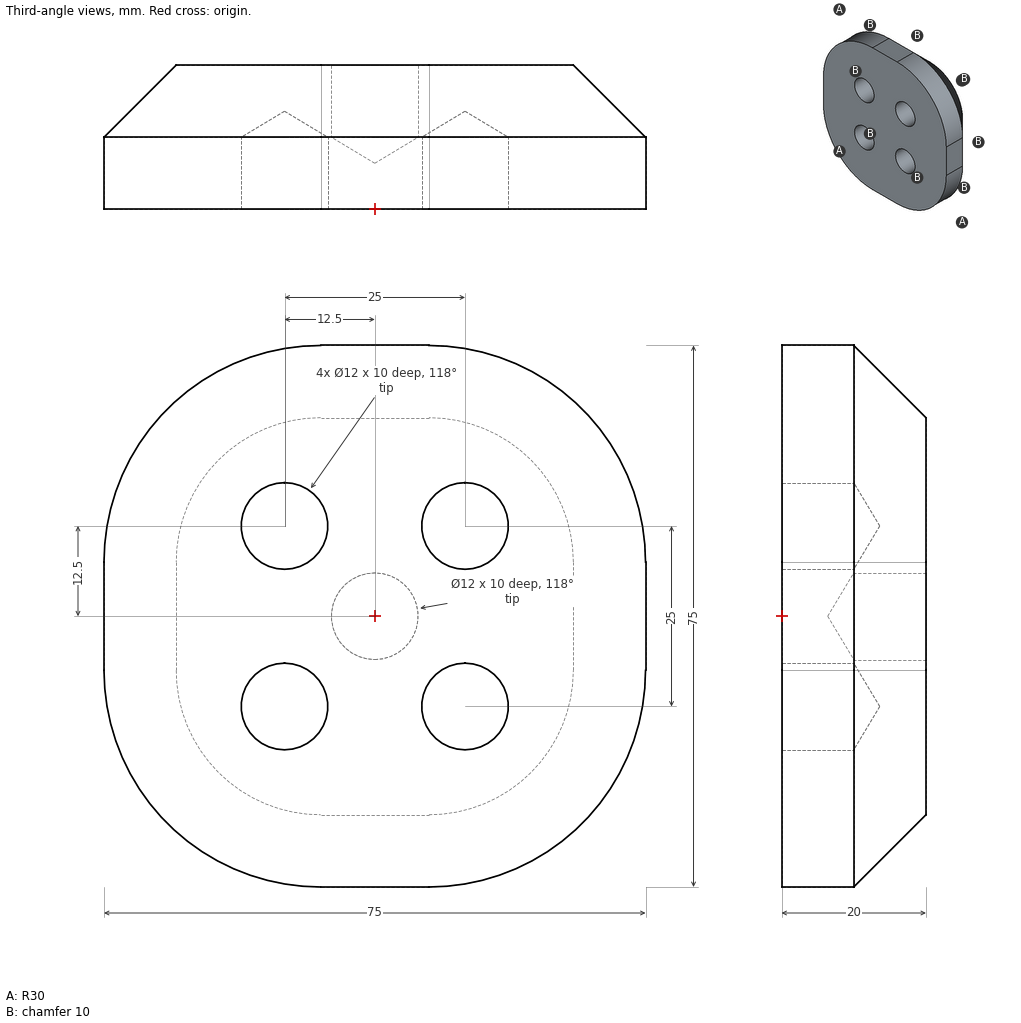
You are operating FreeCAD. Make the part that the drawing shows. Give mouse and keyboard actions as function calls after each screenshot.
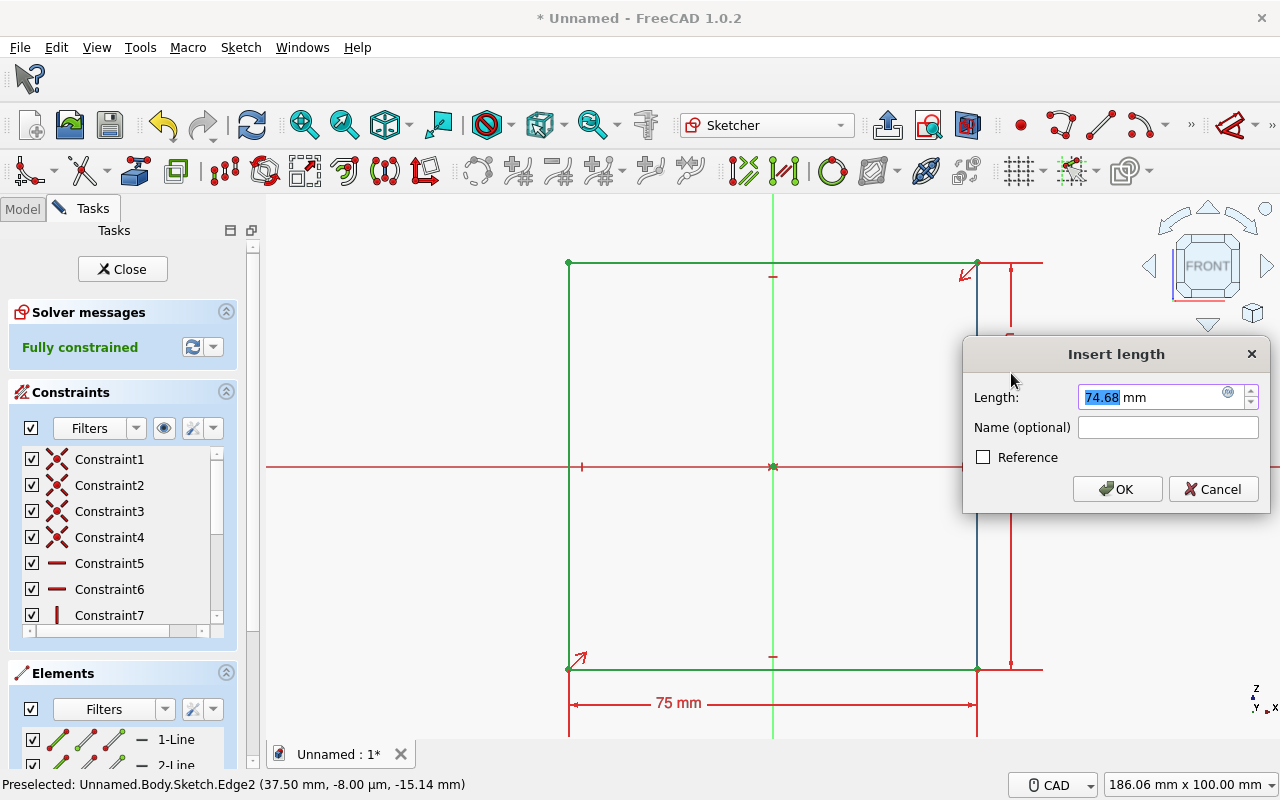
text(75)
key(Return)
key(Escape)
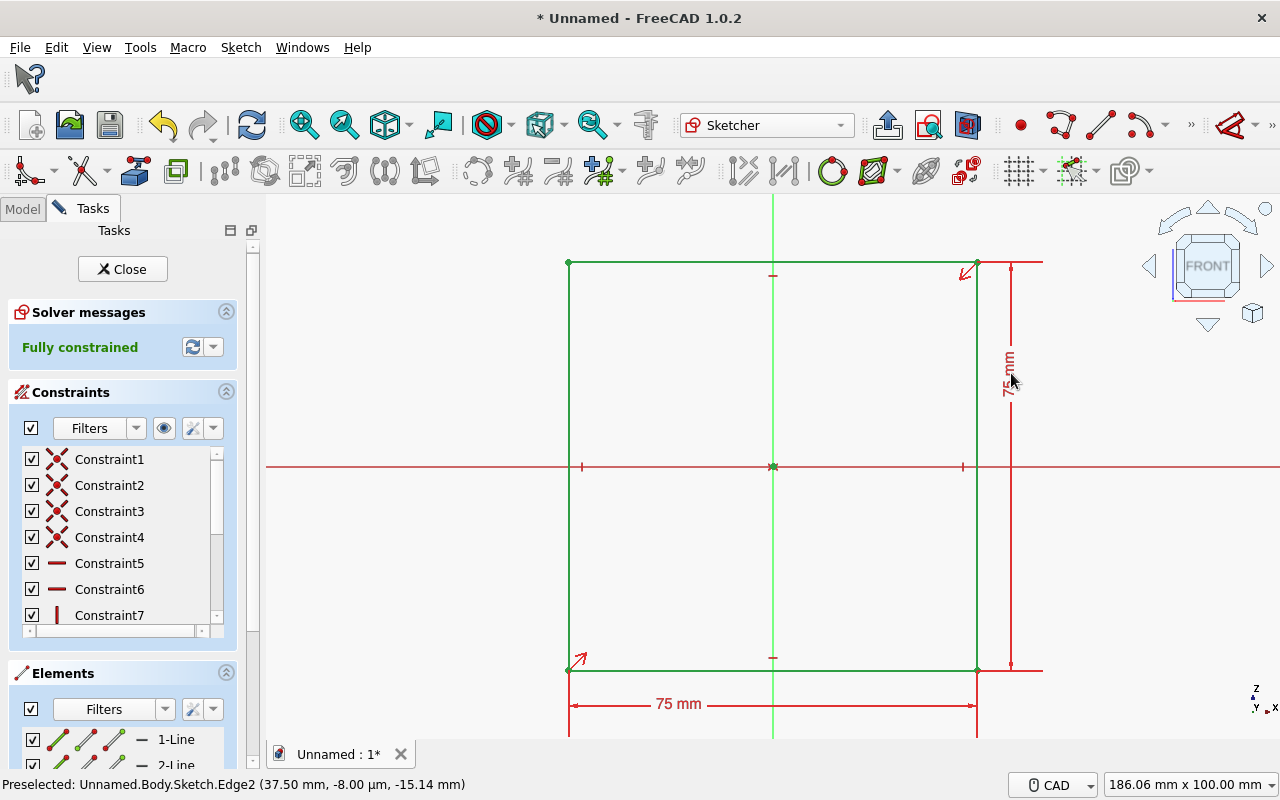
click(123, 269)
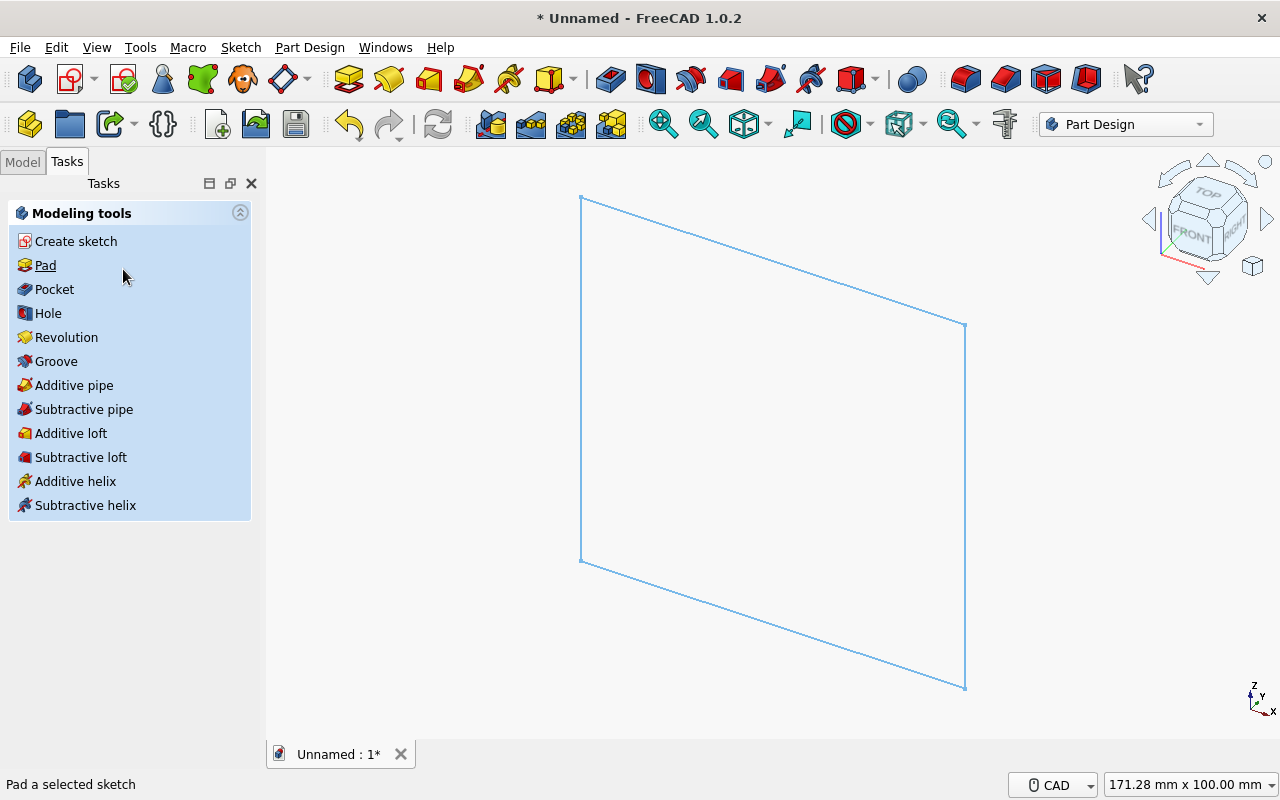
click(350, 80)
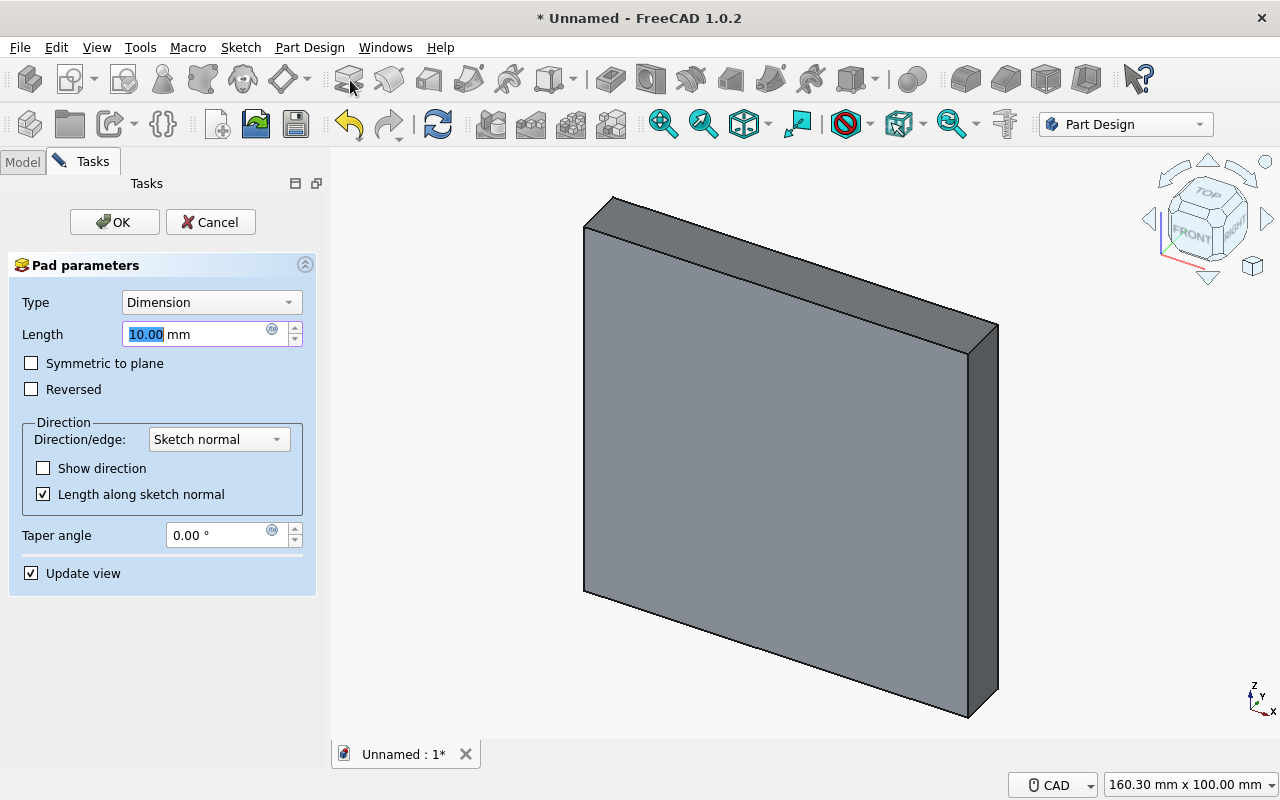
text(20)
key(Tab)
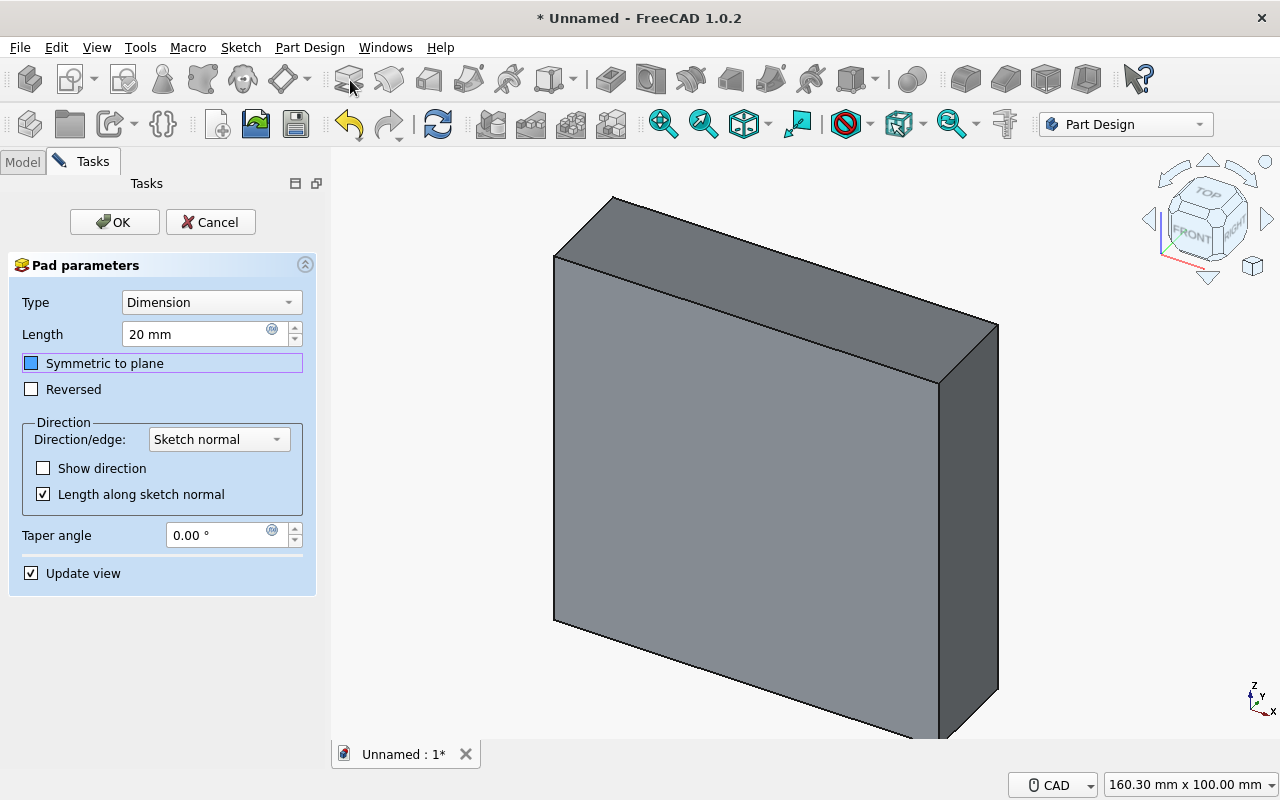
click(30, 389)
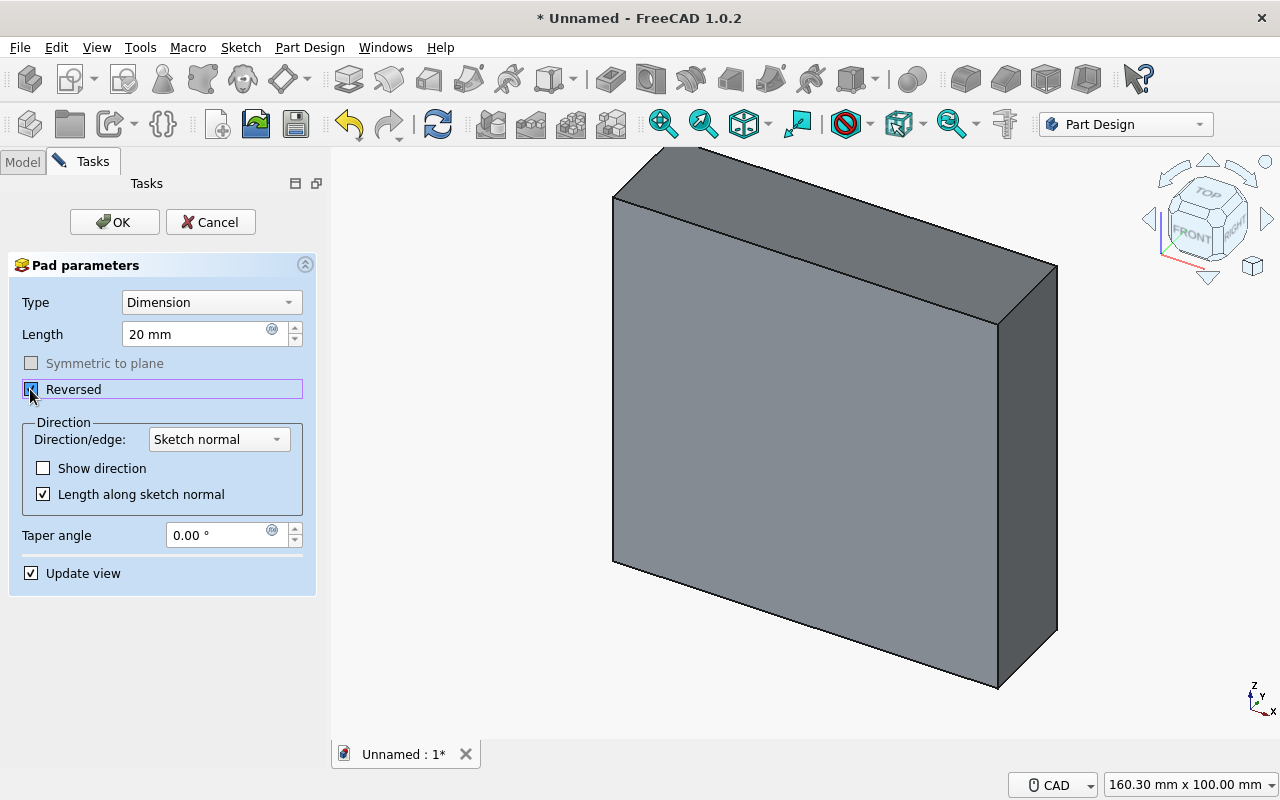
click(115, 222)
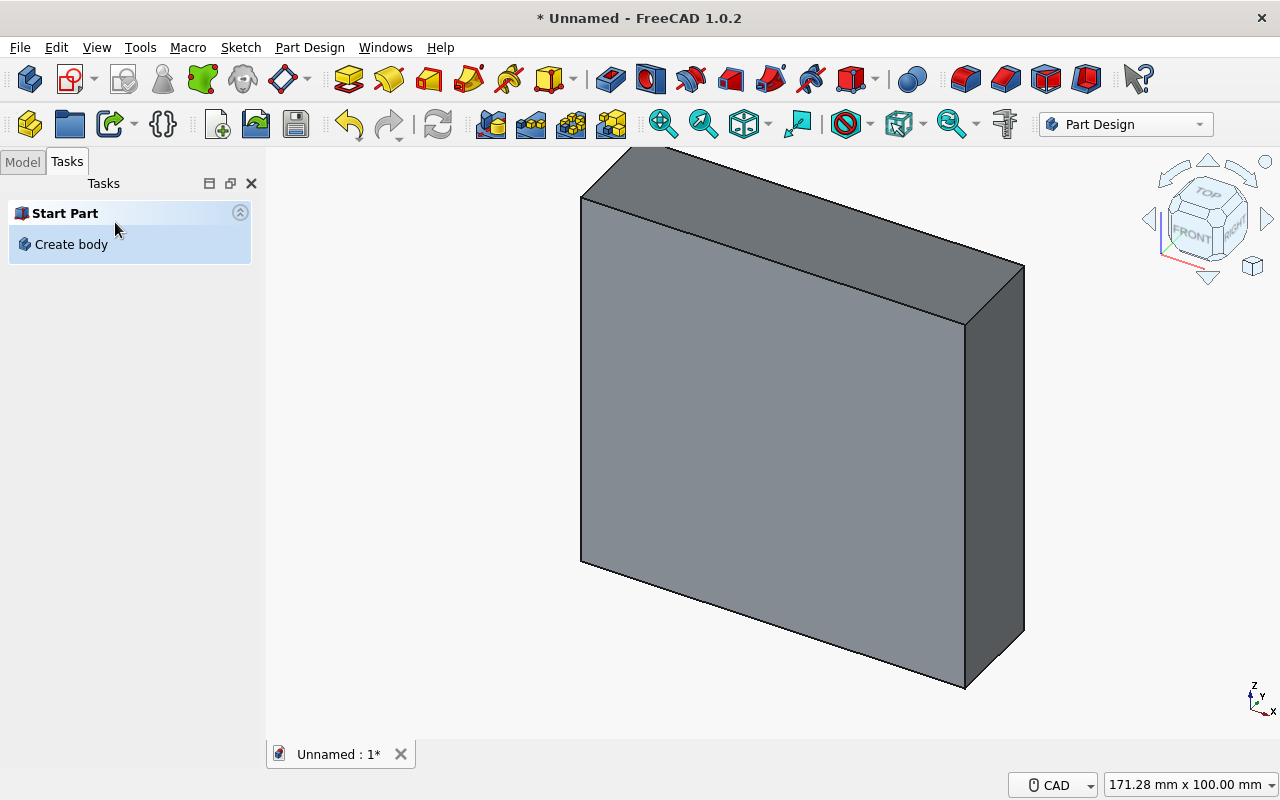
click(664, 124)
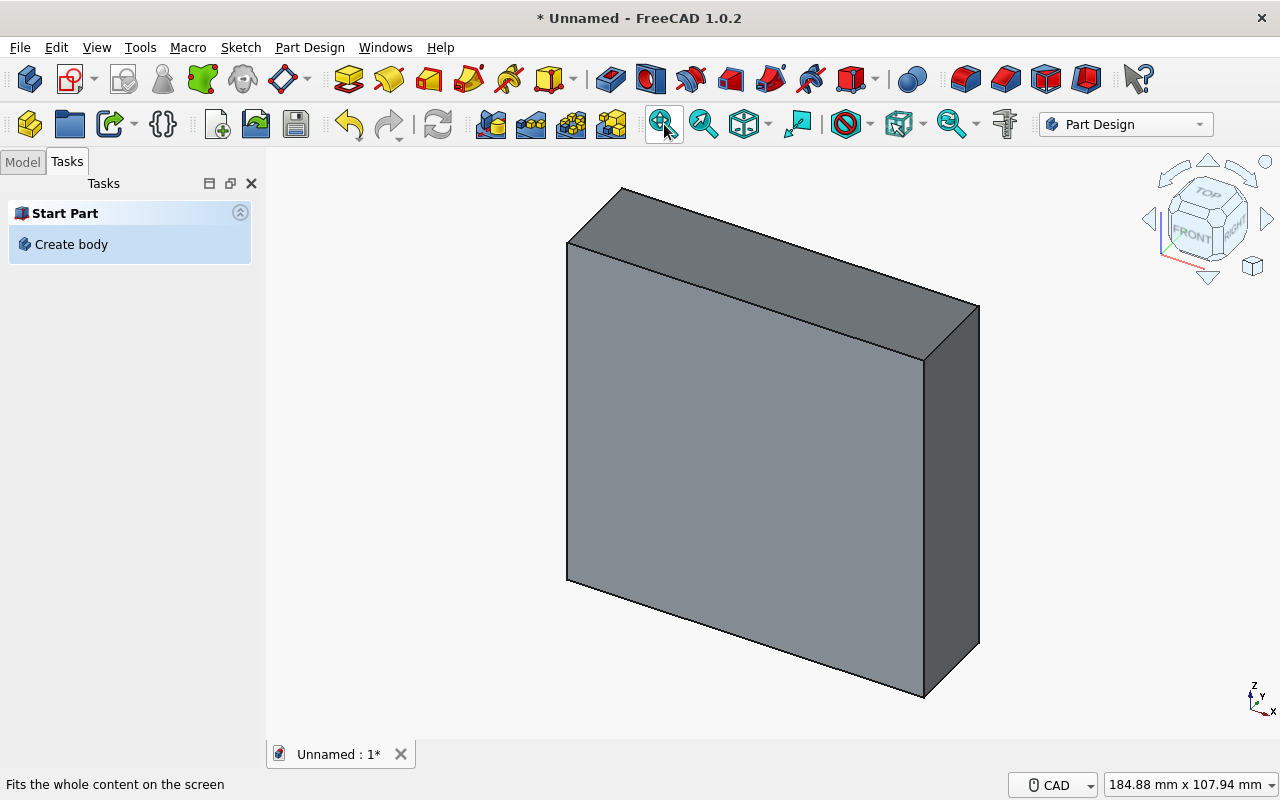
click(951, 333)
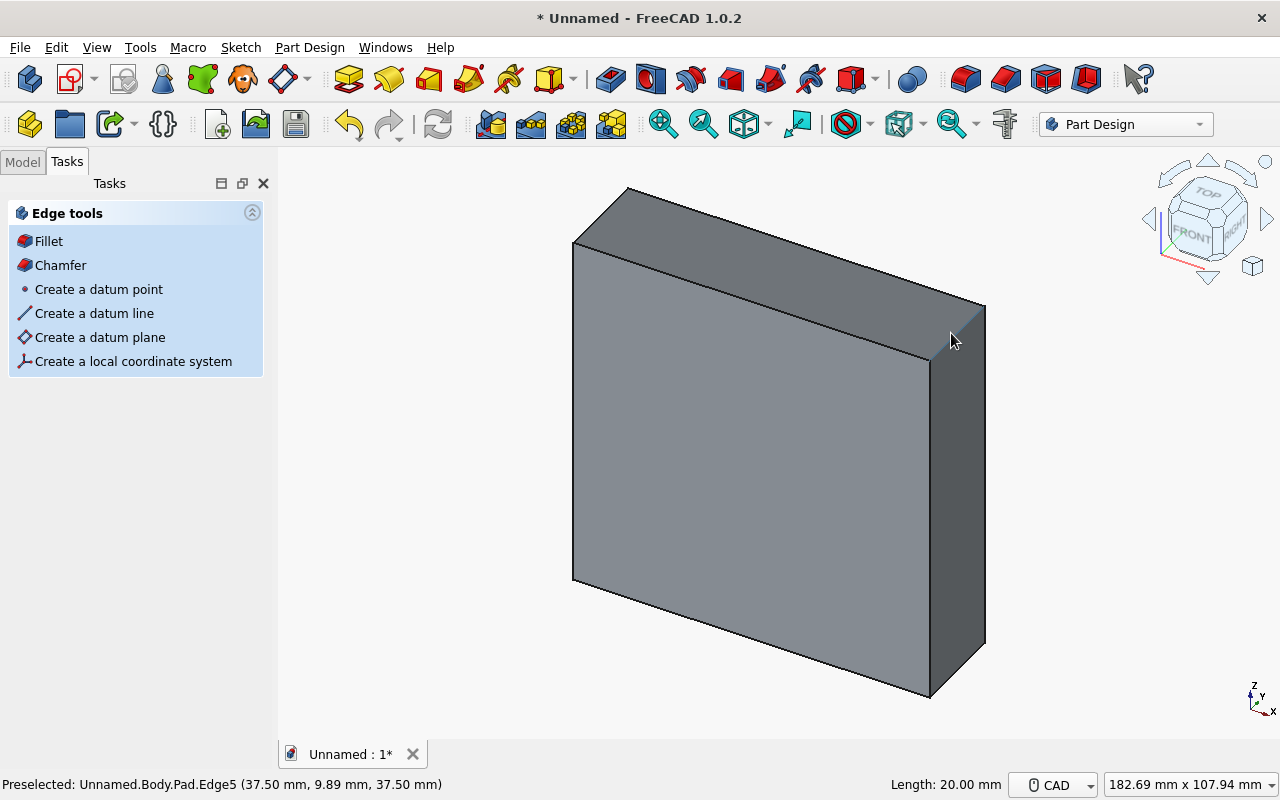
key(0)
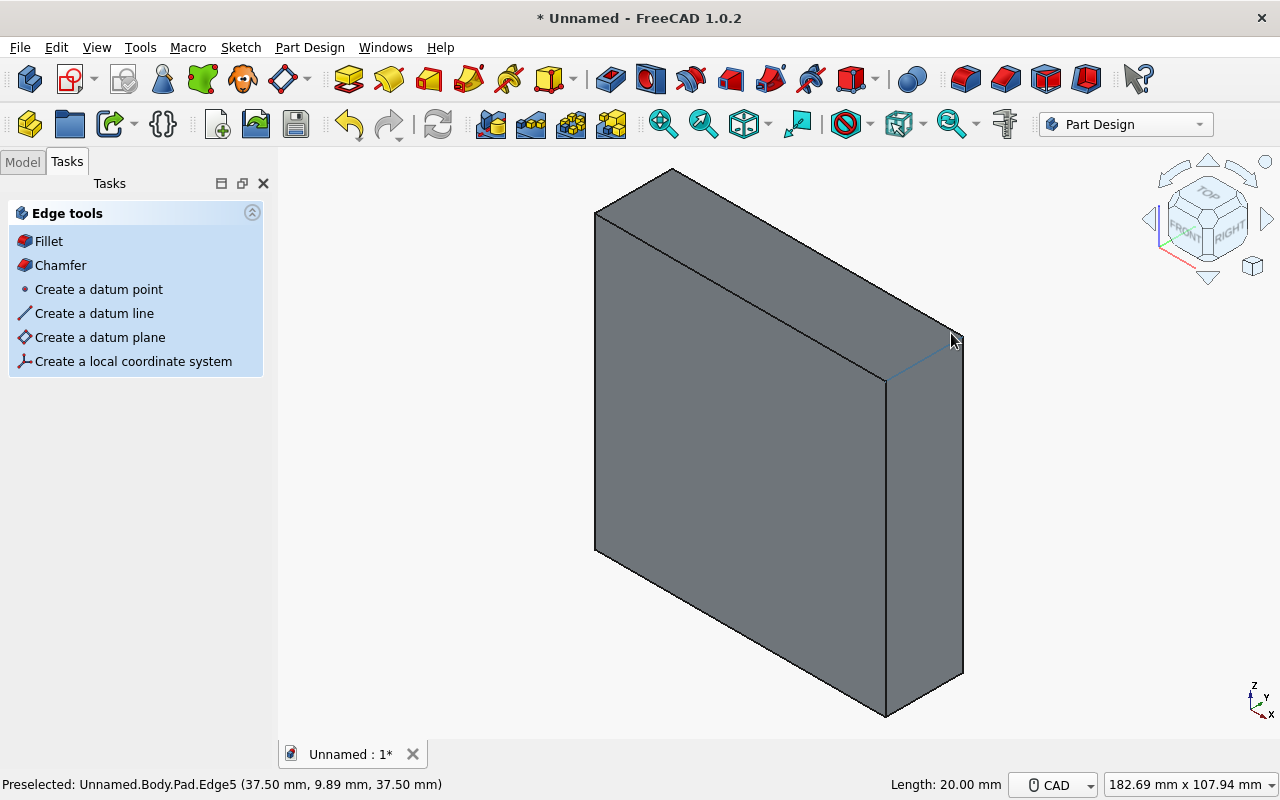
key(2)